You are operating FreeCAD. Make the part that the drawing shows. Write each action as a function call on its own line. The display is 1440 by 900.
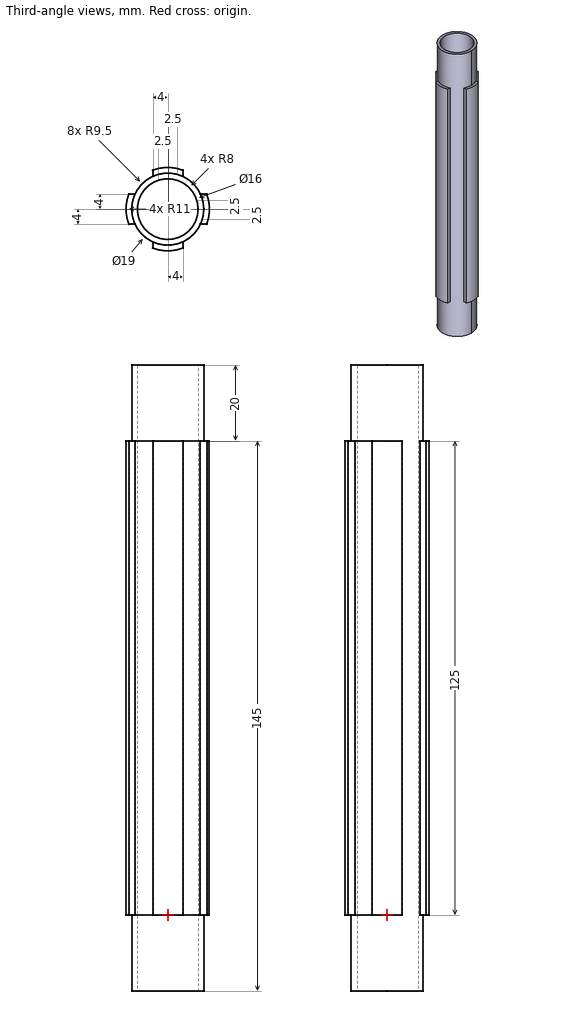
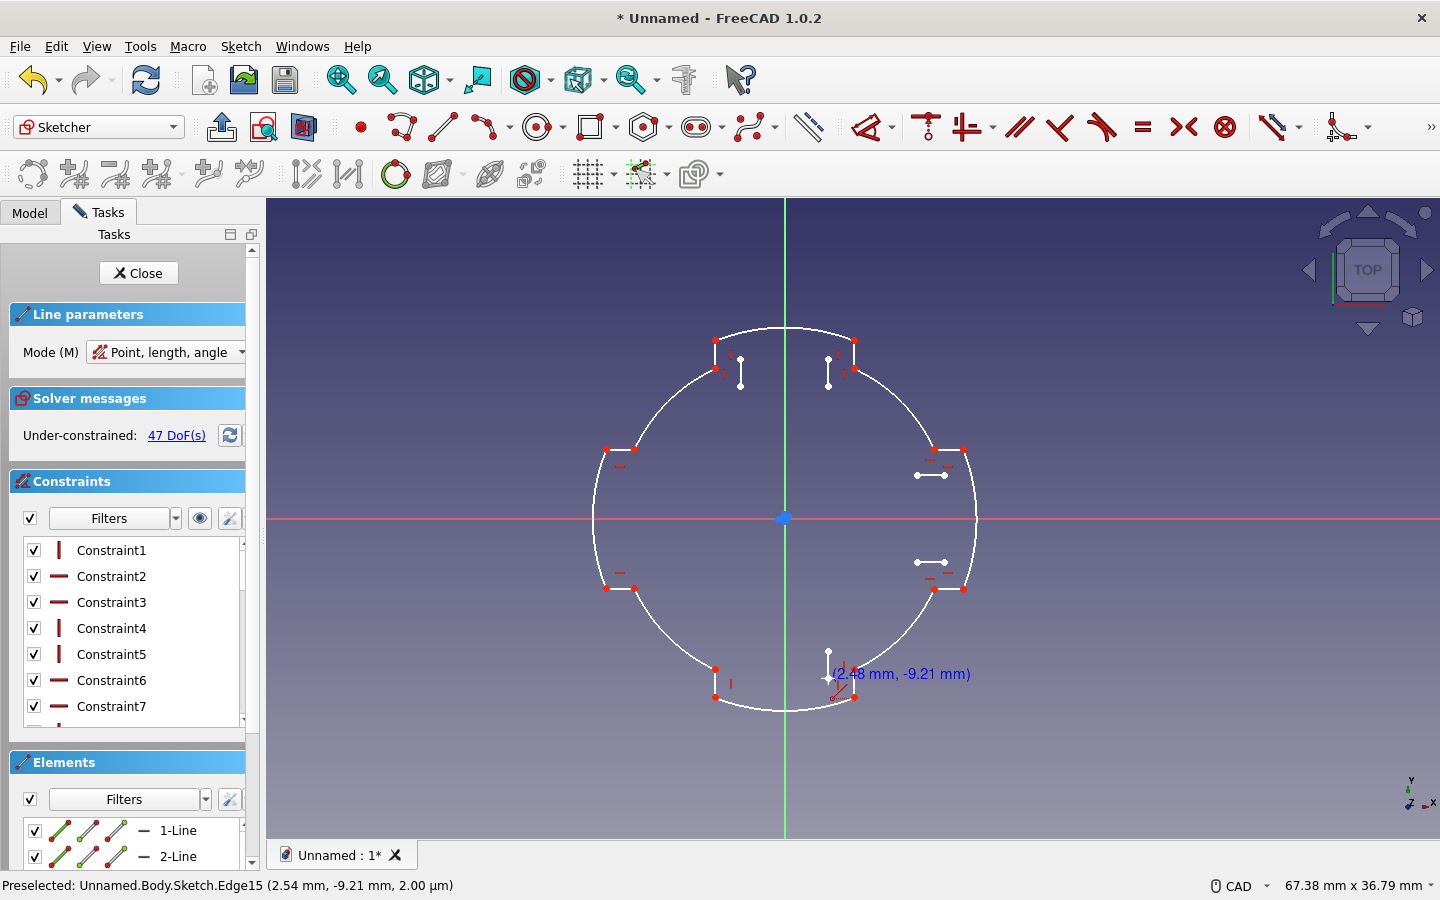
click(741, 678)
click(741, 651)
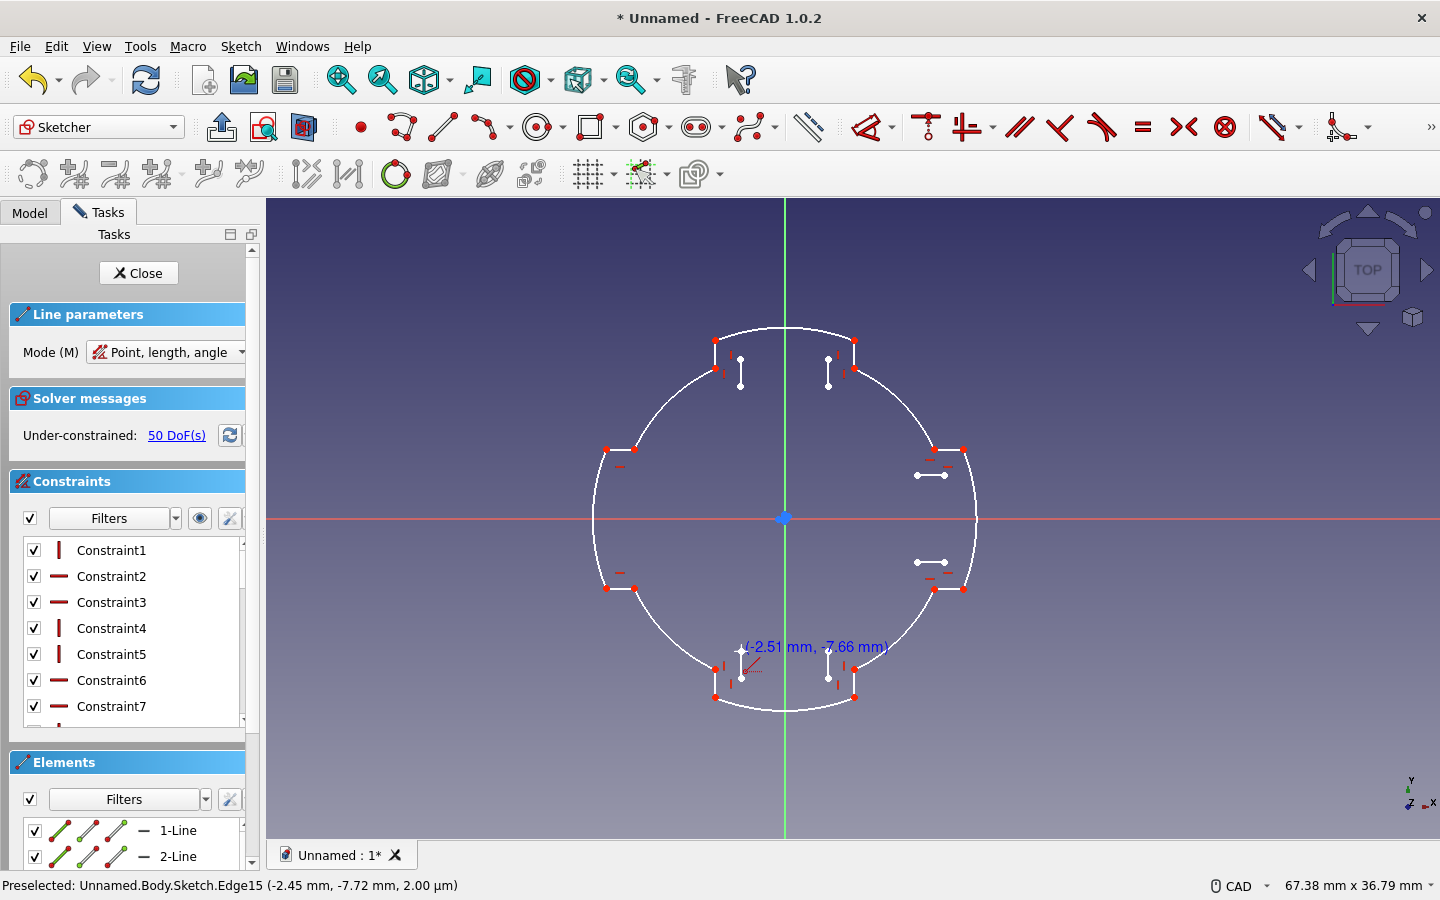
click(652, 562)
click(625, 562)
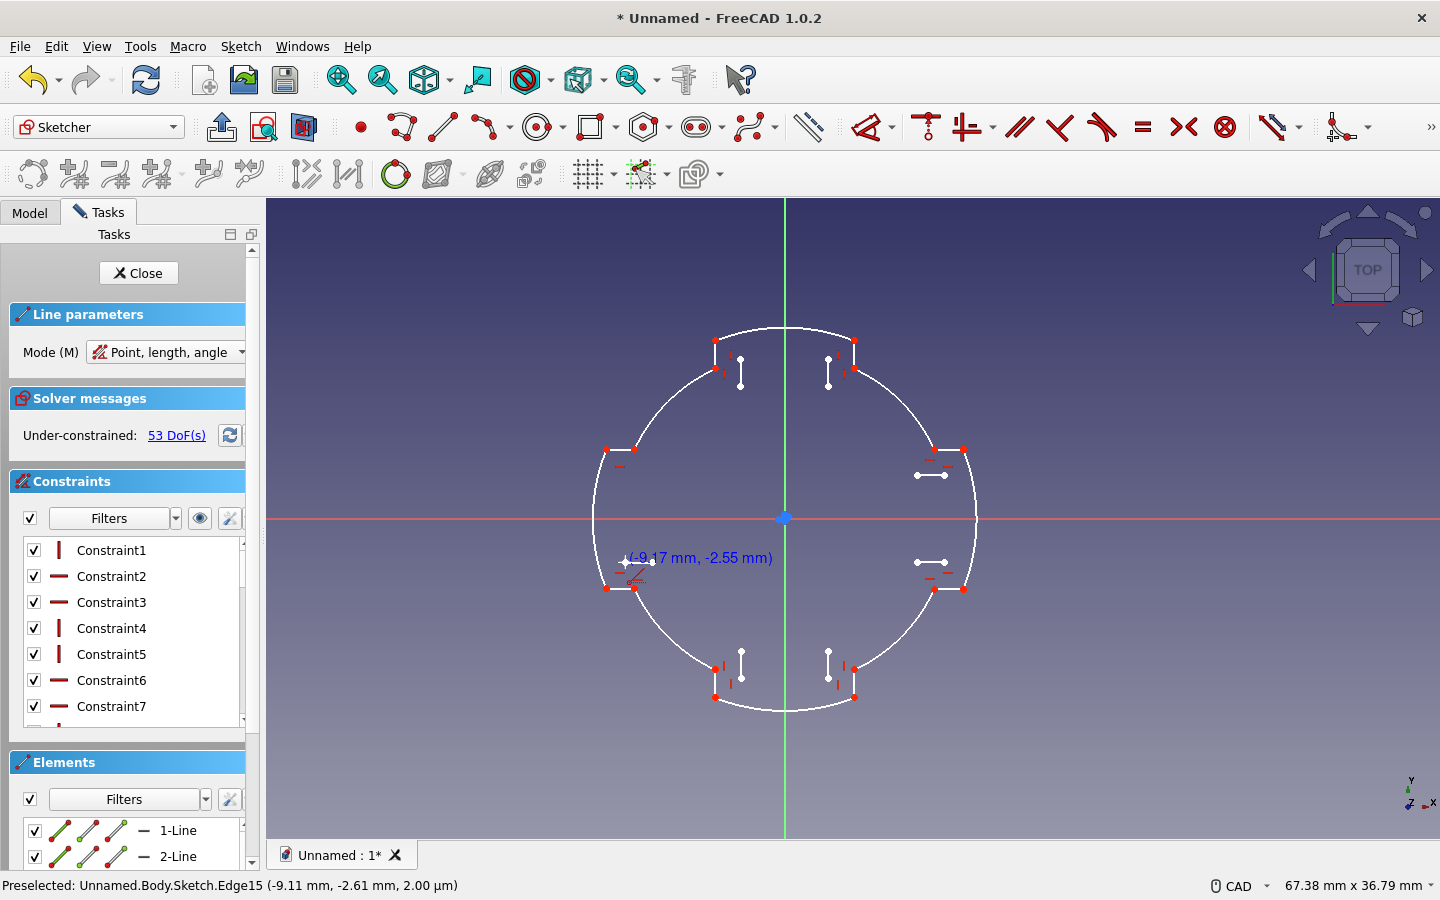
click(625, 475)
click(652, 475)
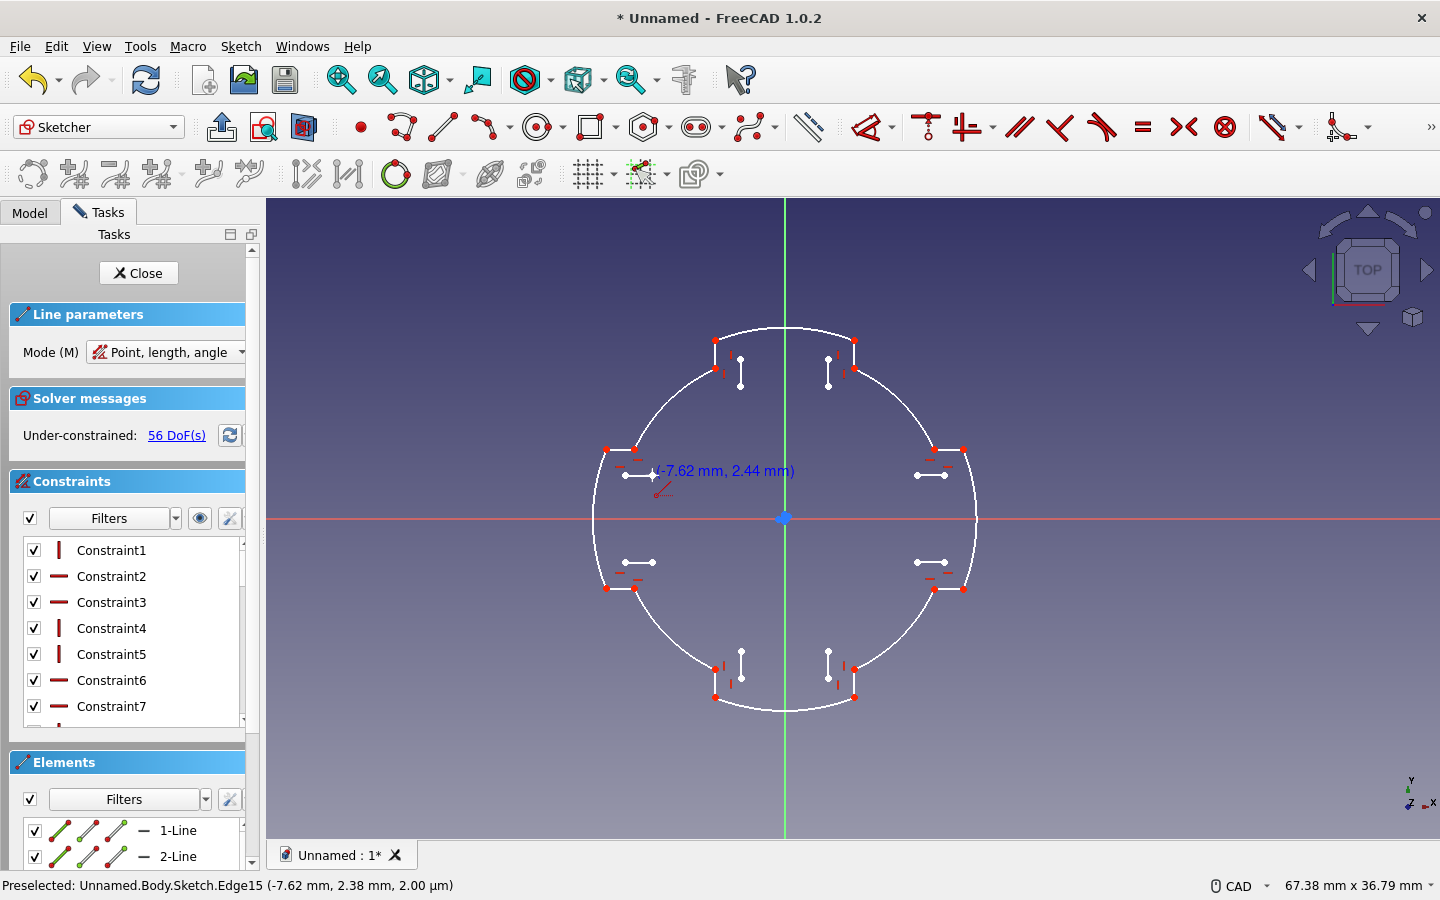
click(484, 128)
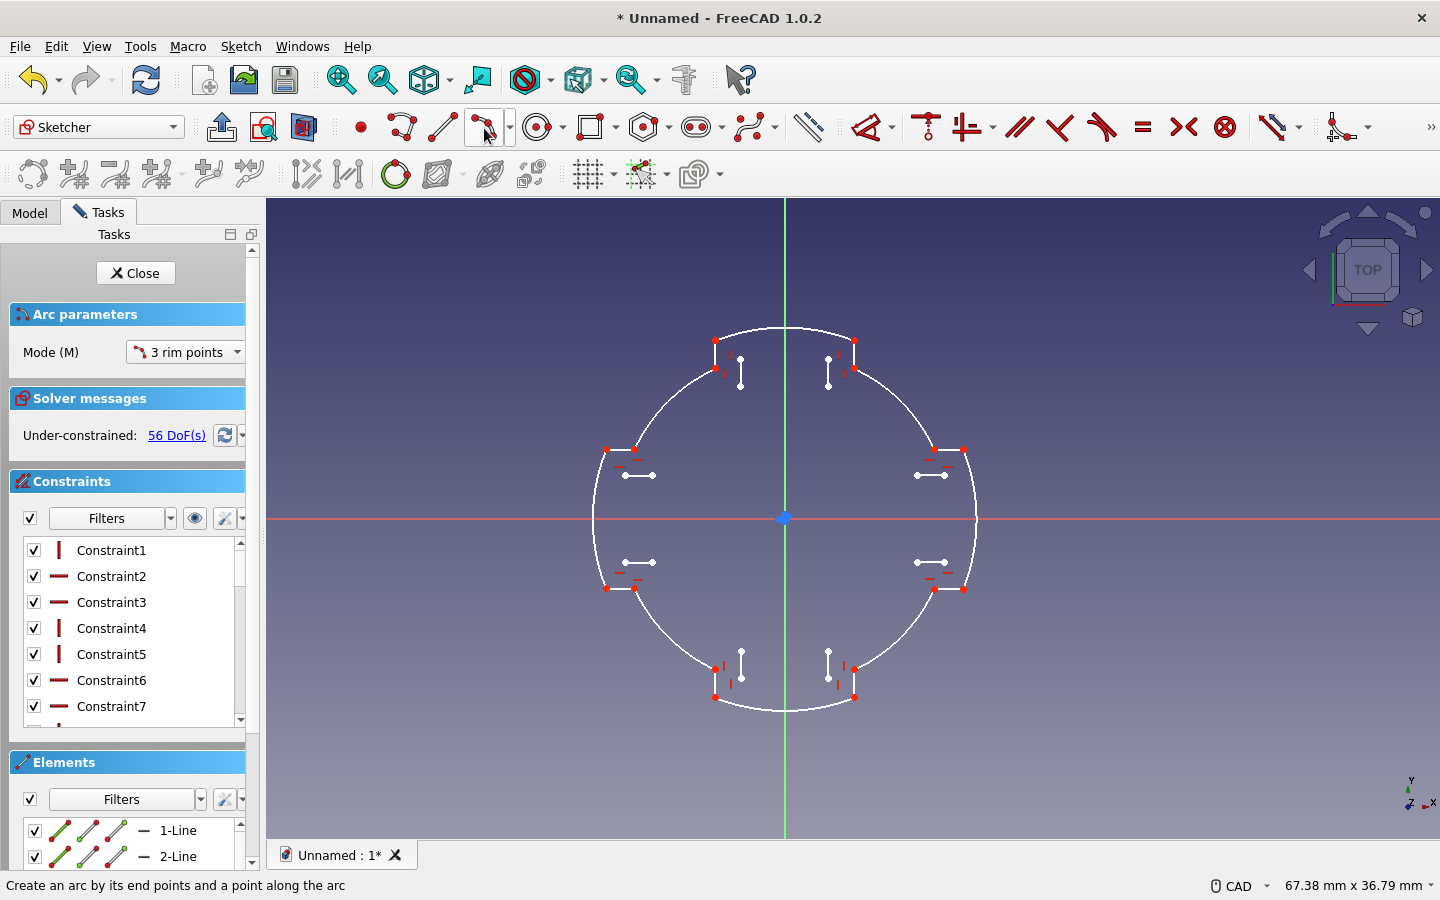
click(741, 359)
click(828, 359)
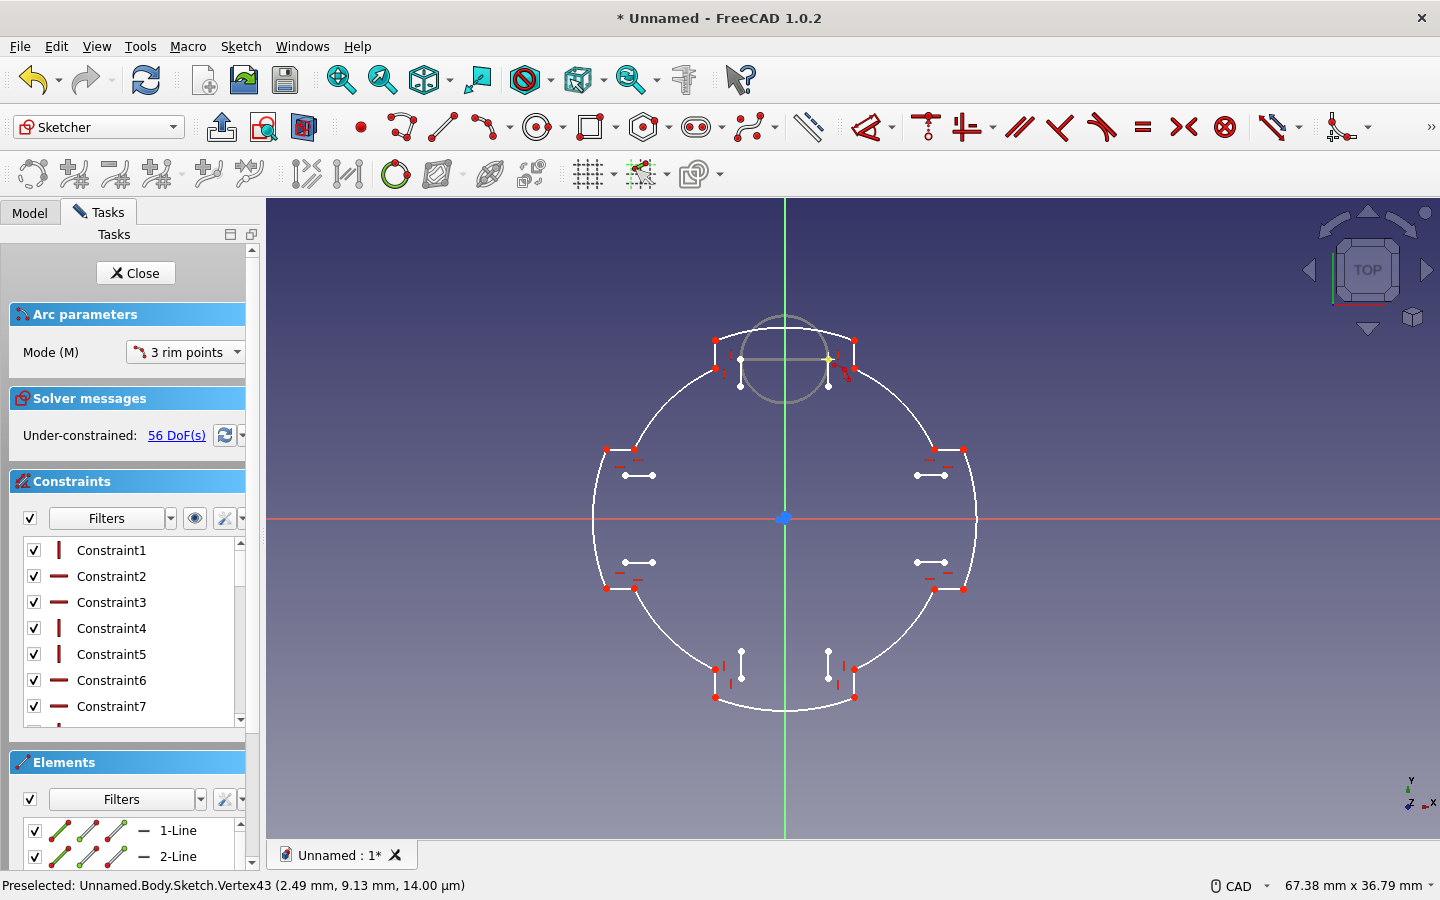
scroll(794, 353, up, 6)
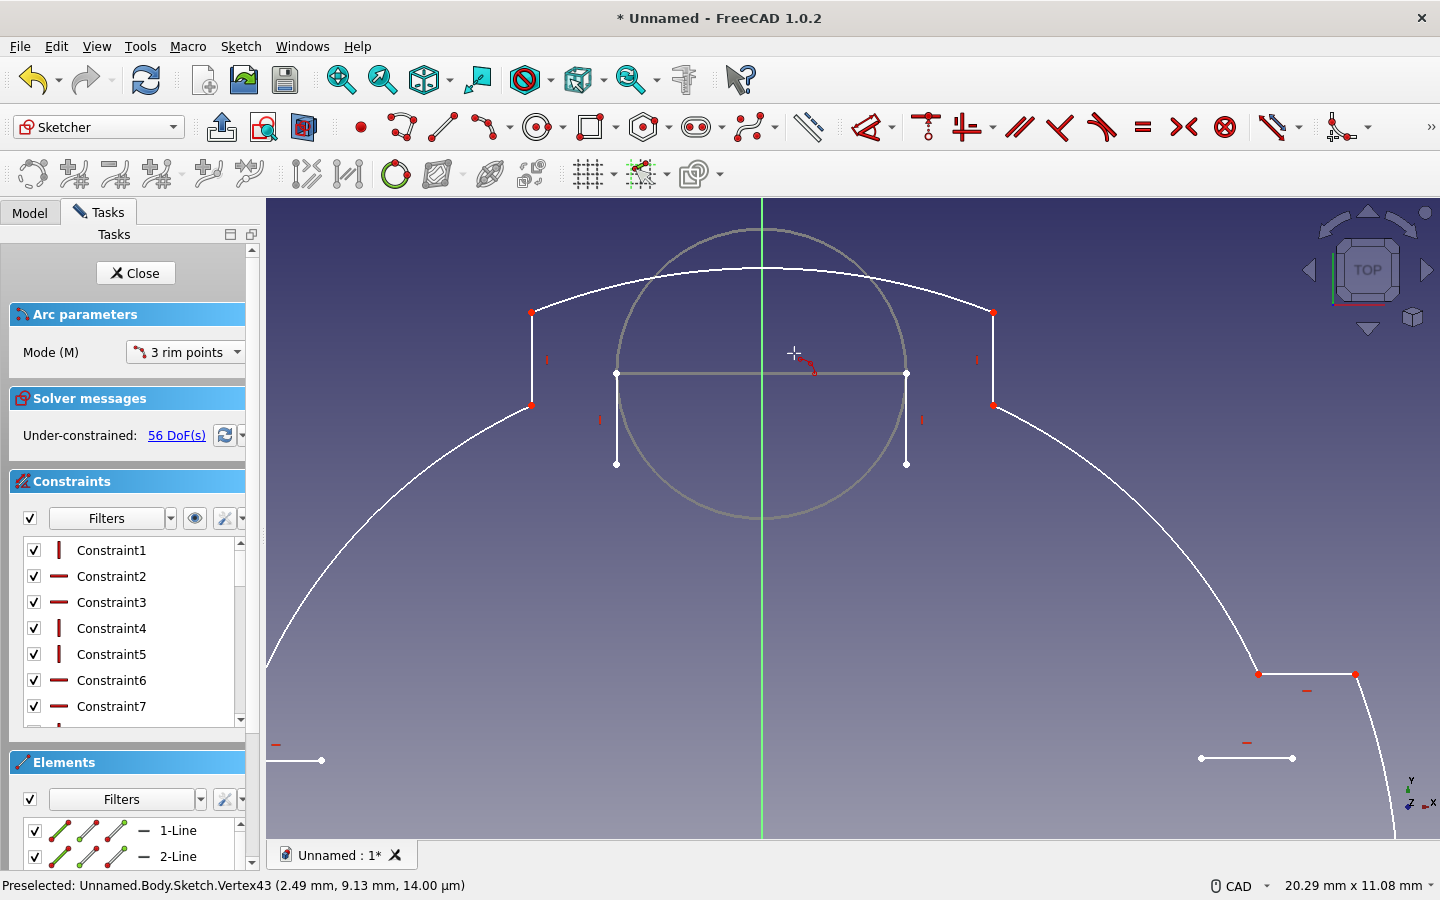
click(791, 353)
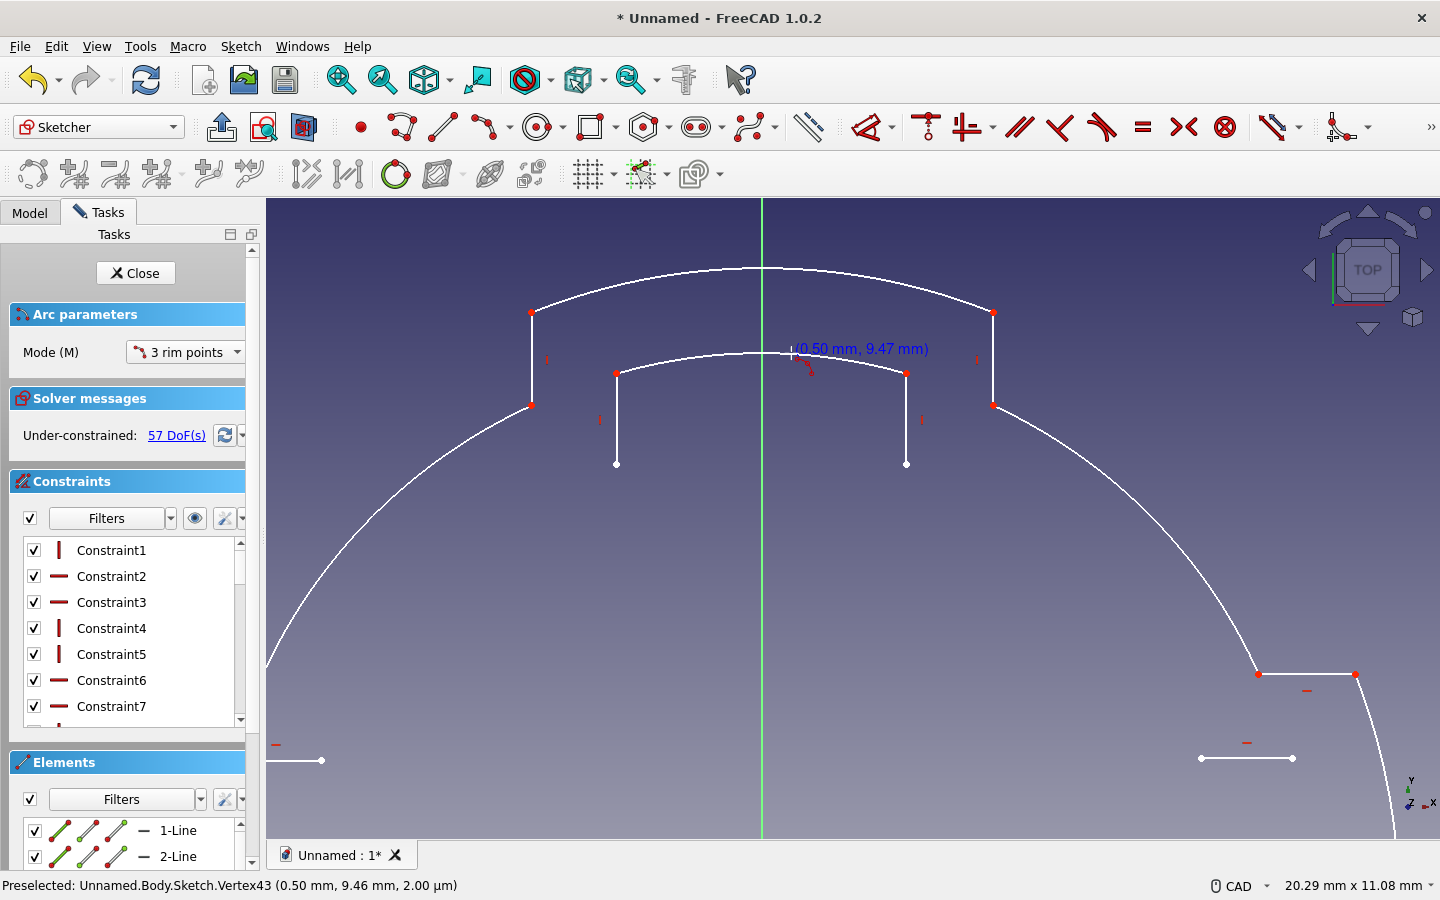
click(906, 465)
click(1202, 758)
click(1089, 575)